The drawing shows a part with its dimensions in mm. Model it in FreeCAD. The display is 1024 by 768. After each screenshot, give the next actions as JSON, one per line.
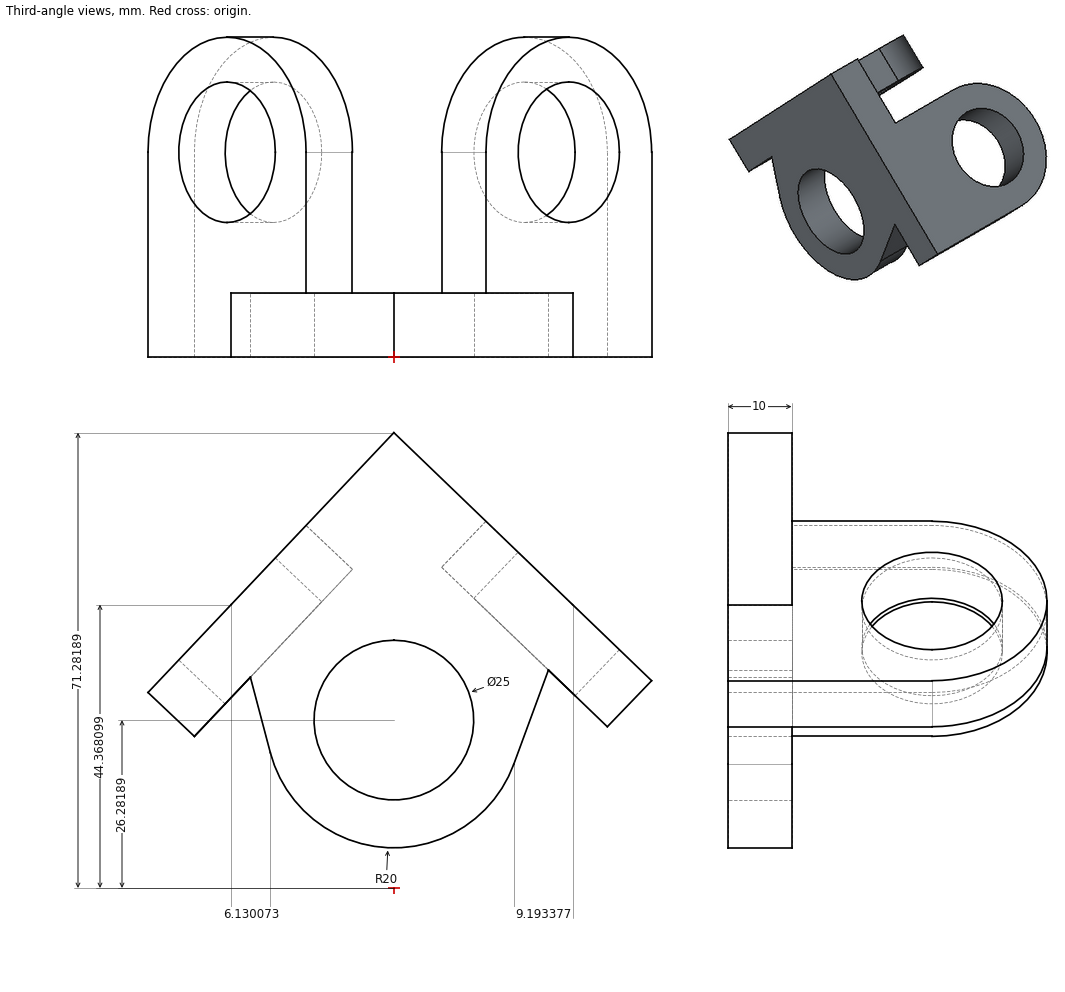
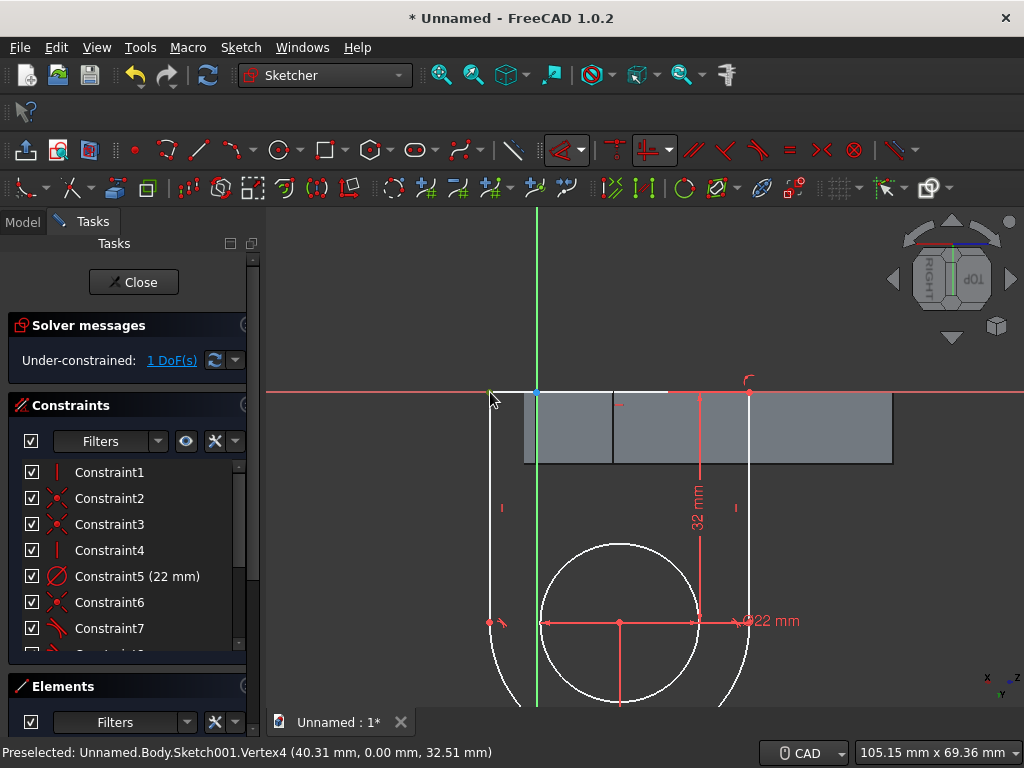
{"action": "left_click", "coordinate": [584, 150]}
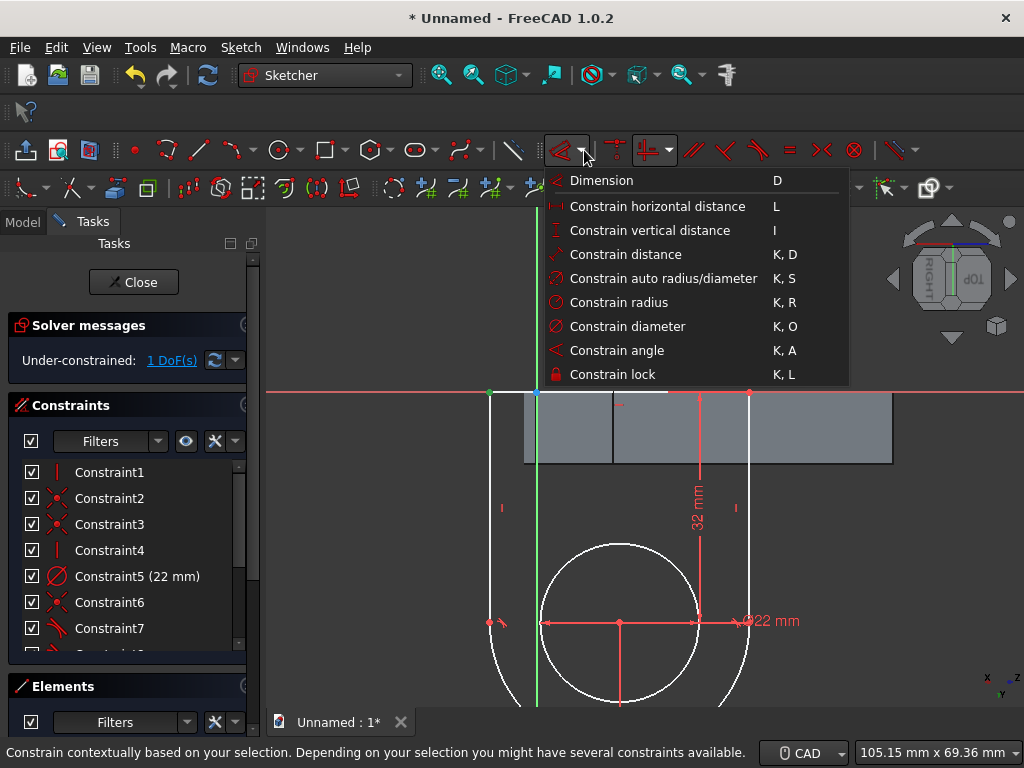
{"action": "left_click", "coordinate": [697, 206]}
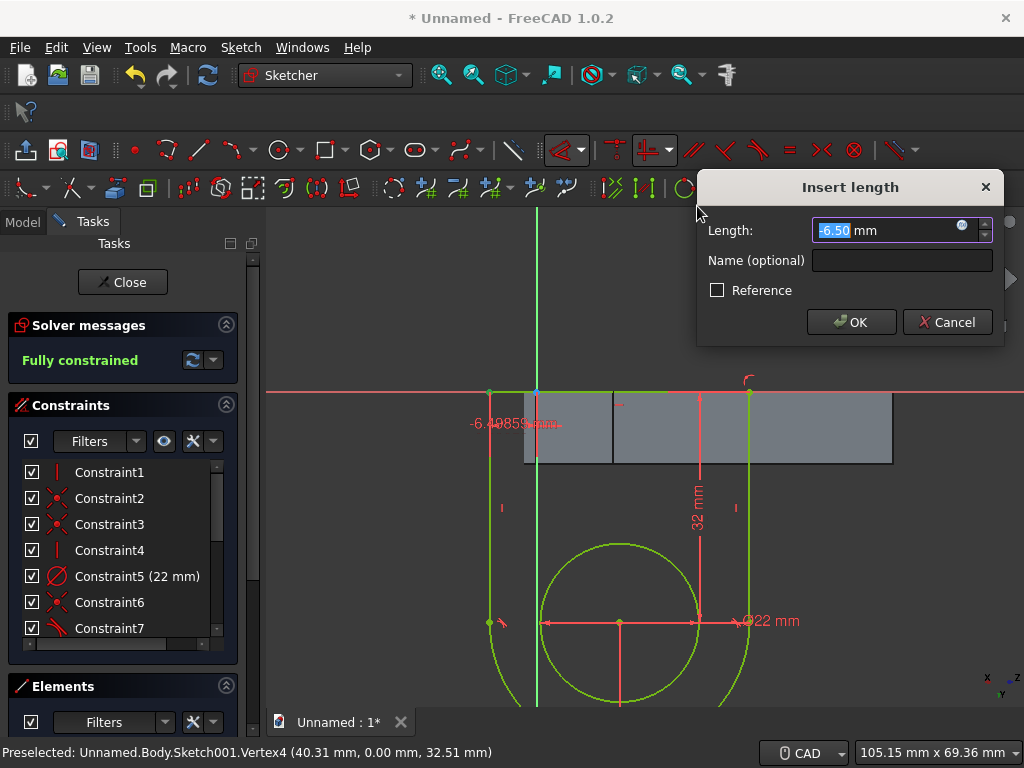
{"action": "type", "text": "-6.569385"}
{"action": "key", "text": "Return"}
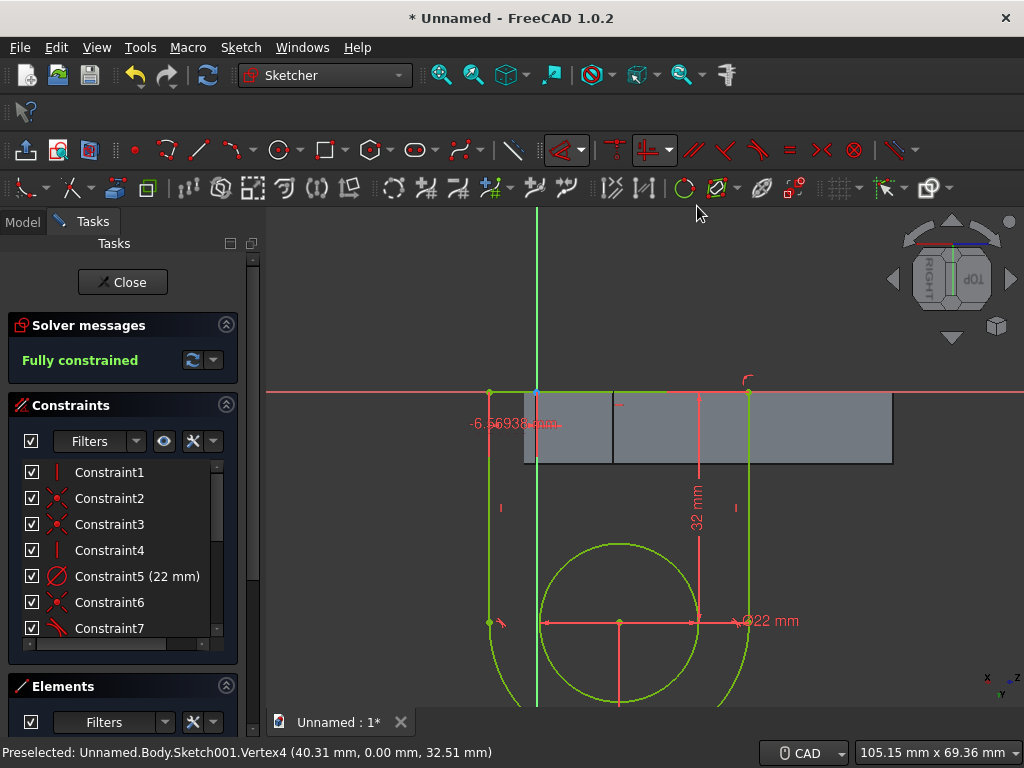
{"action": "left_click", "coordinate": [123, 282]}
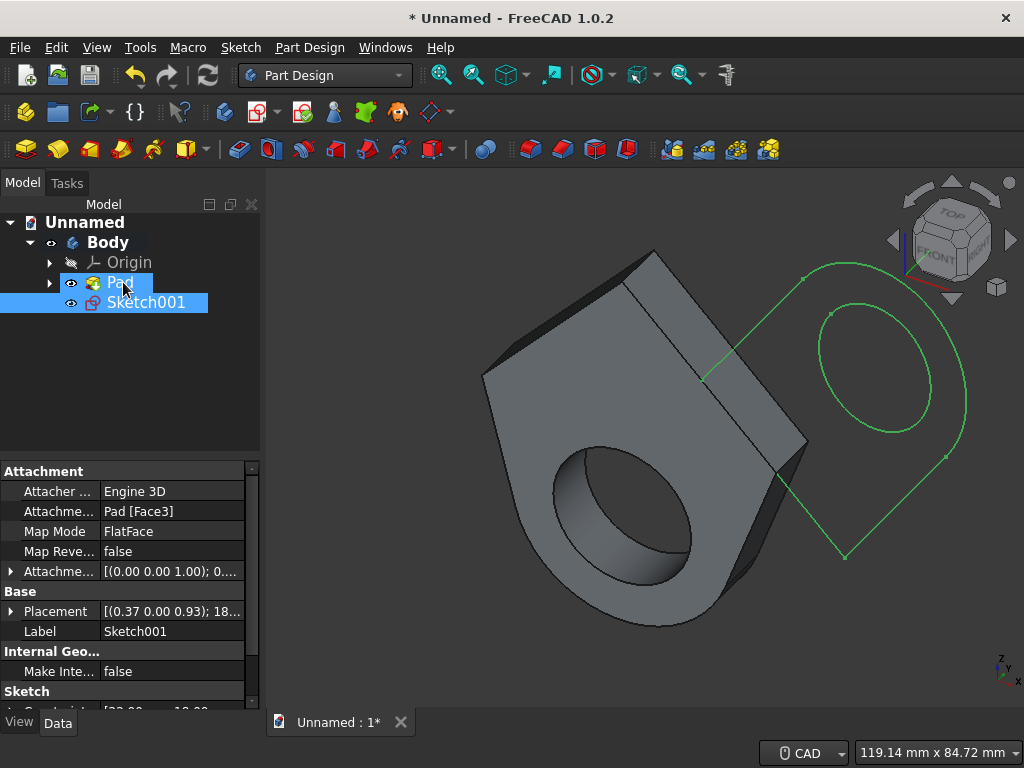
{"action": "left_click", "coordinate": [26, 150]}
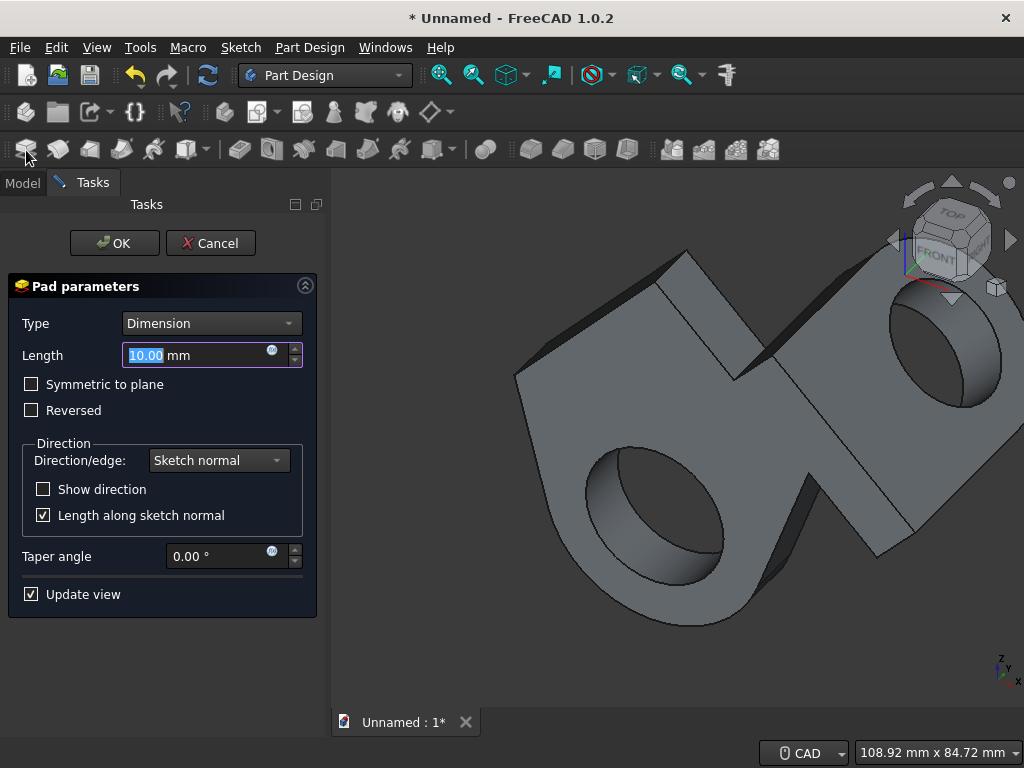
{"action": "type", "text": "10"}
{"action": "key", "text": "Tab"}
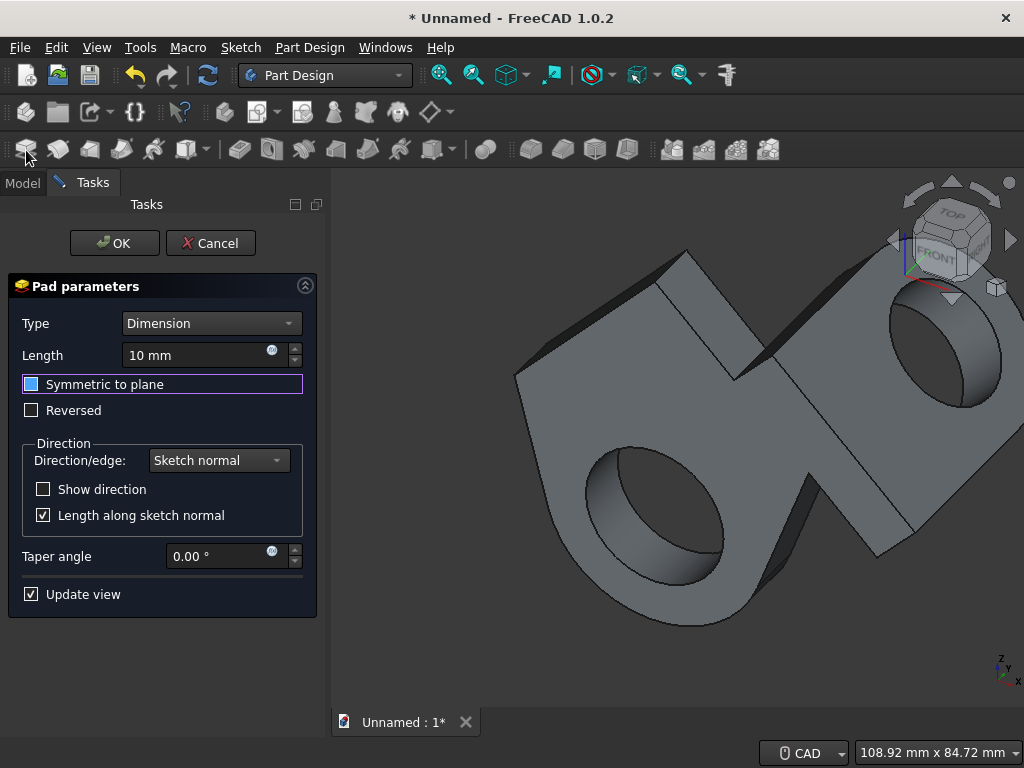
{"action": "left_click", "coordinate": [30, 410]}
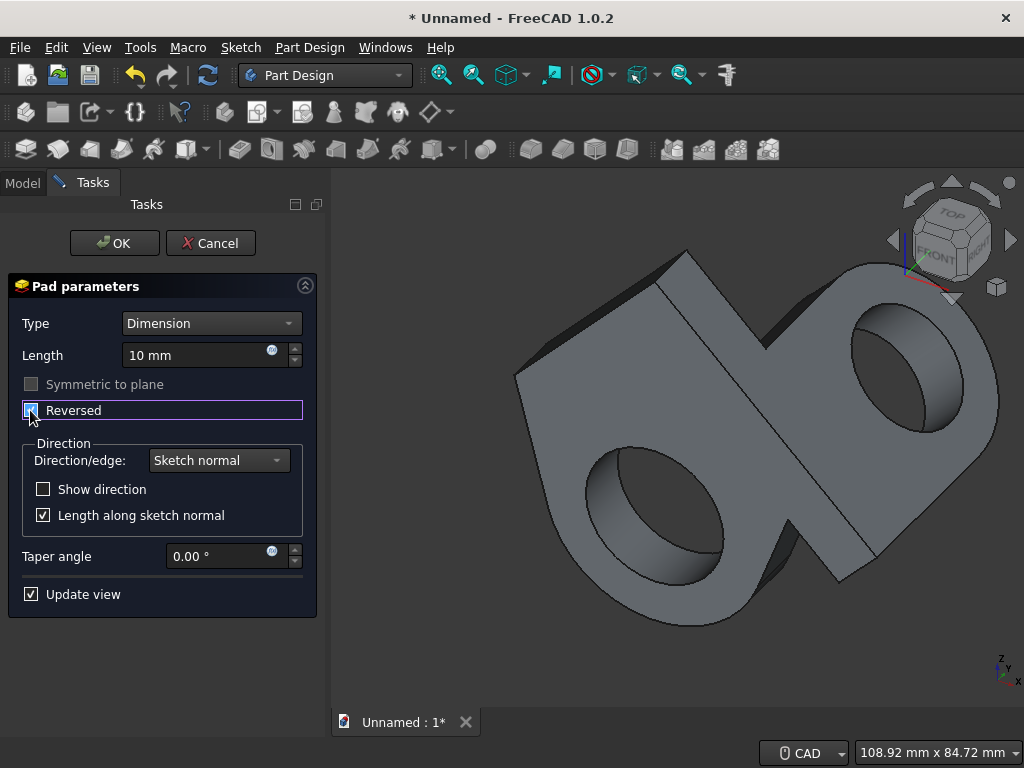
{"action": "left_click", "coordinate": [115, 243]}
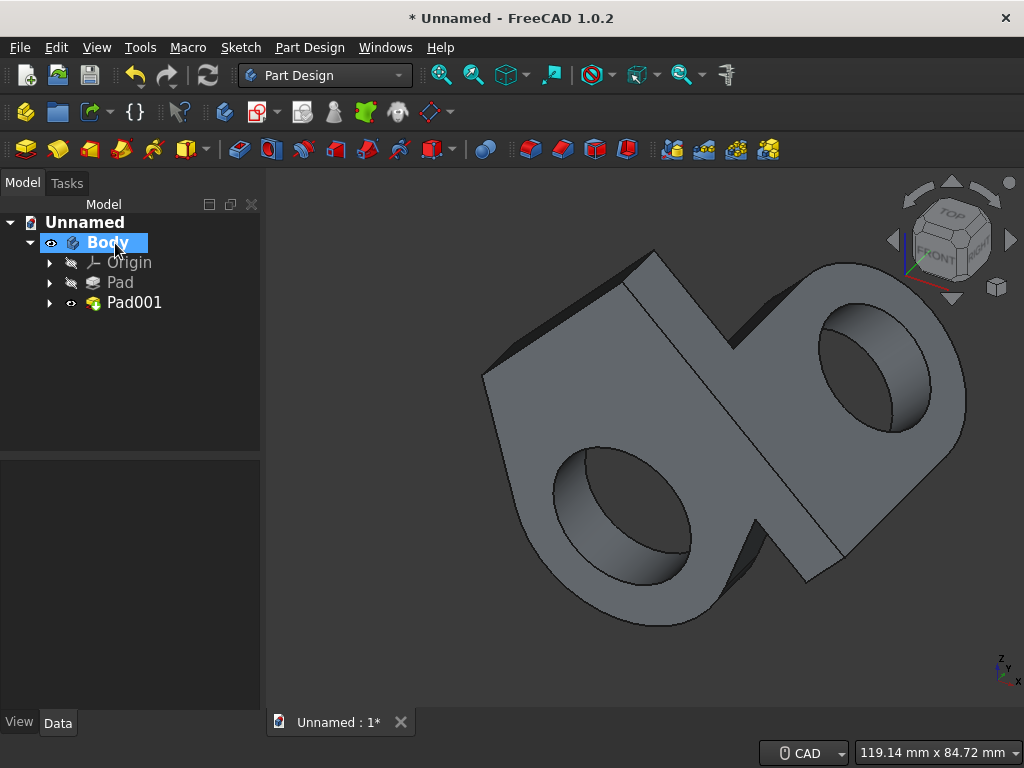
{"action": "left_click", "coordinate": [442, 76]}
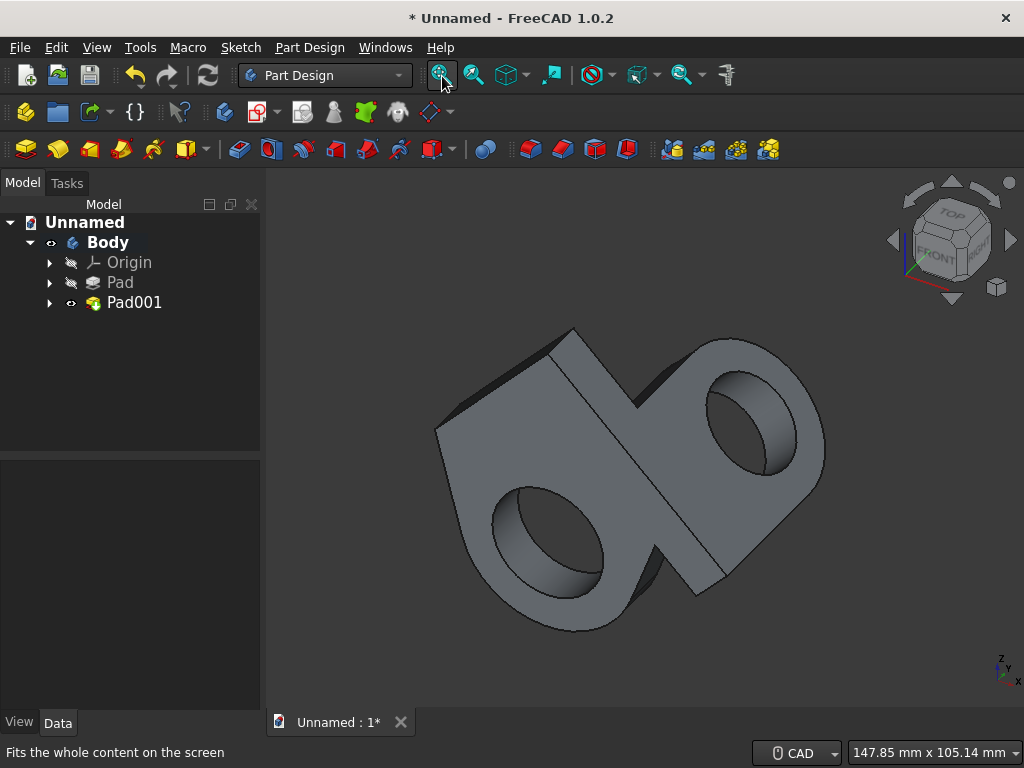
{"action": "key", "text": "6"}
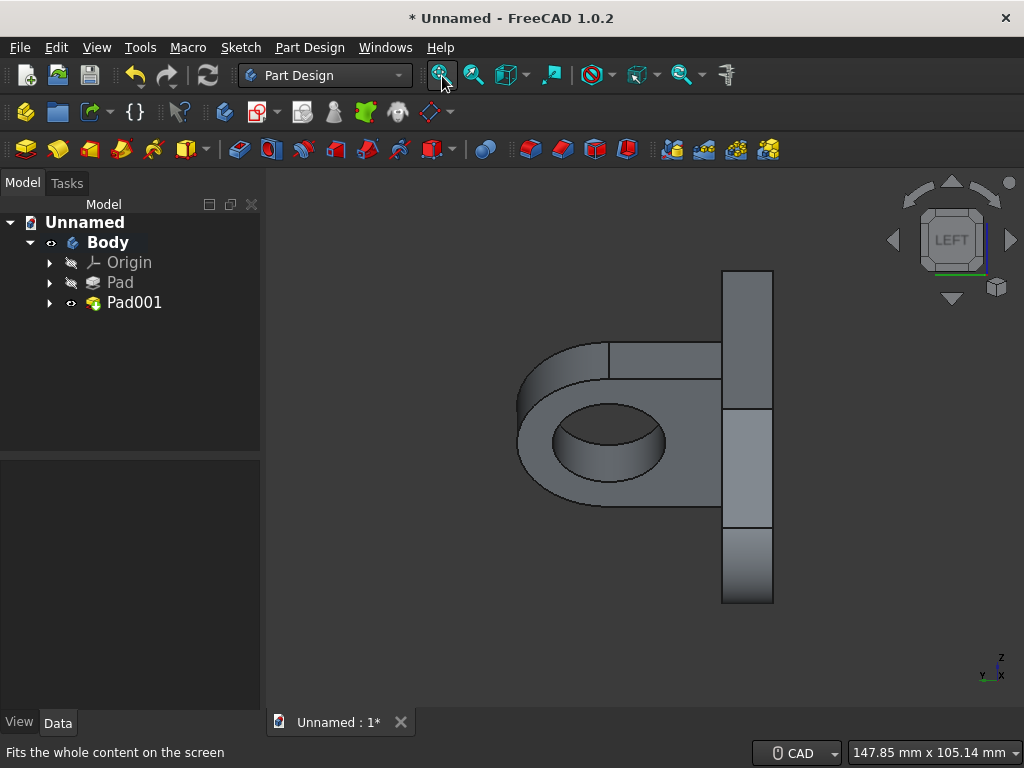
{"action": "left_click", "coordinate": [748, 300]}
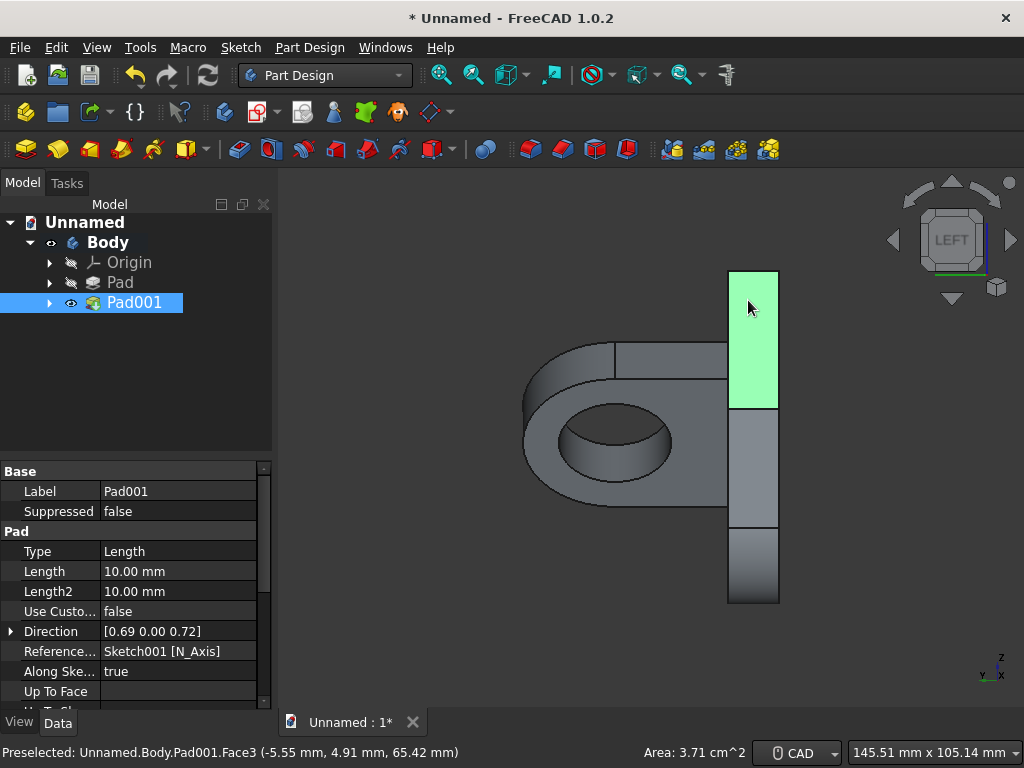
{"action": "left_click", "coordinate": [258, 112]}